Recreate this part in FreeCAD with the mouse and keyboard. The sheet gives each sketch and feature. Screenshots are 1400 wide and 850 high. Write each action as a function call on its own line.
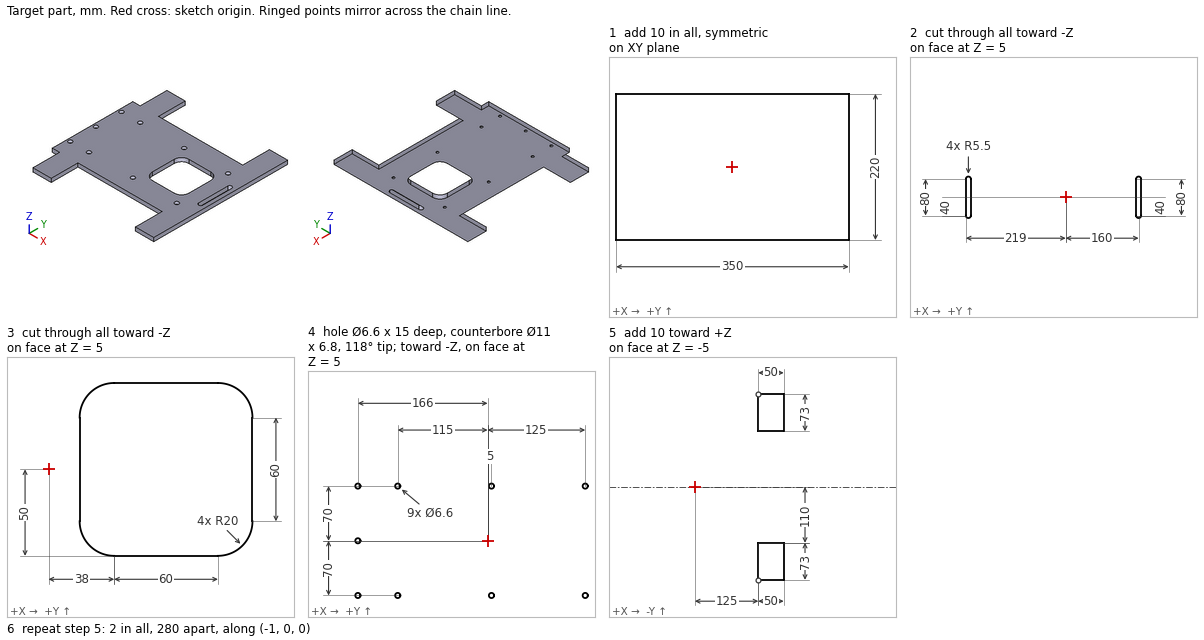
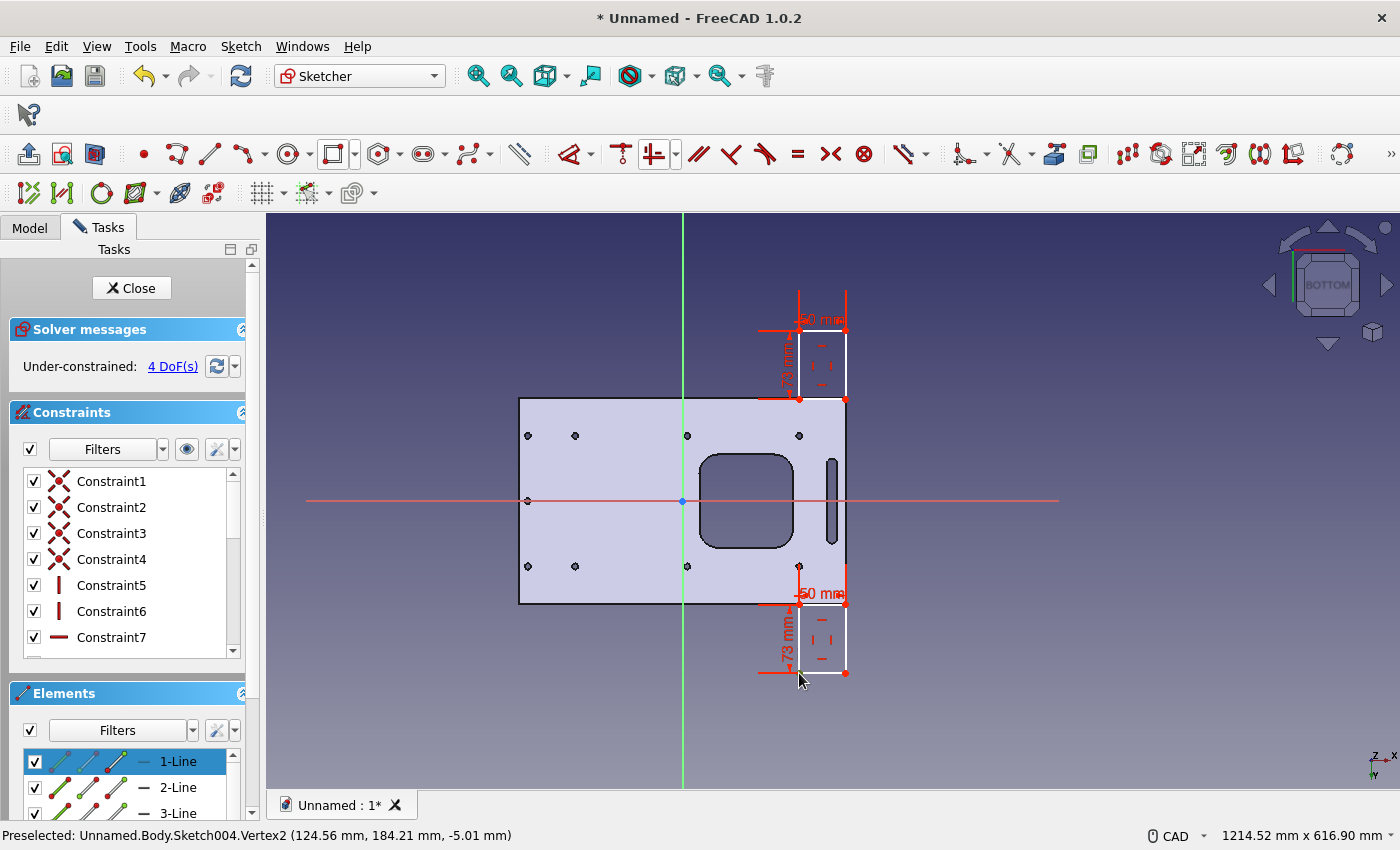
click(799, 331)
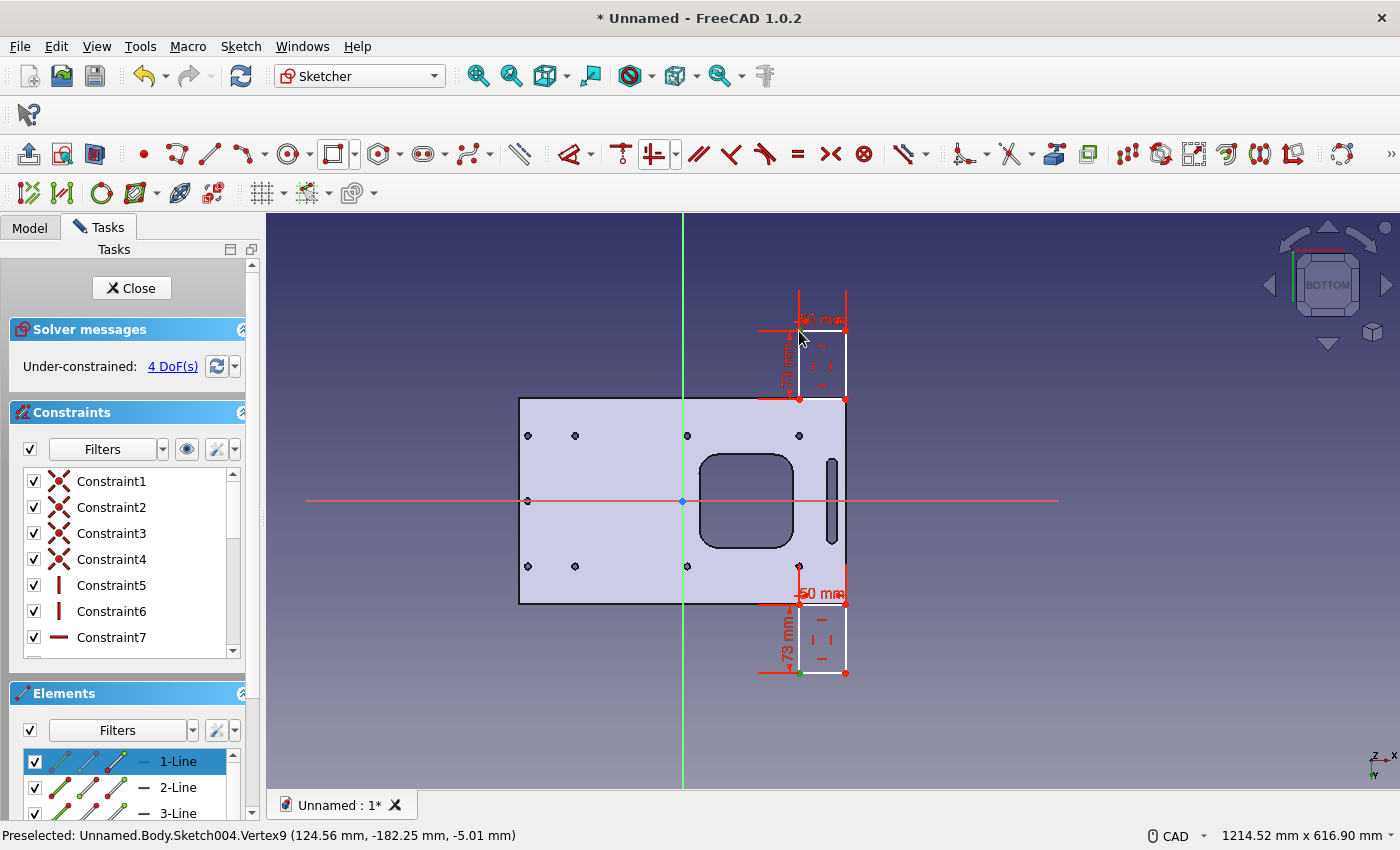
click(361, 501)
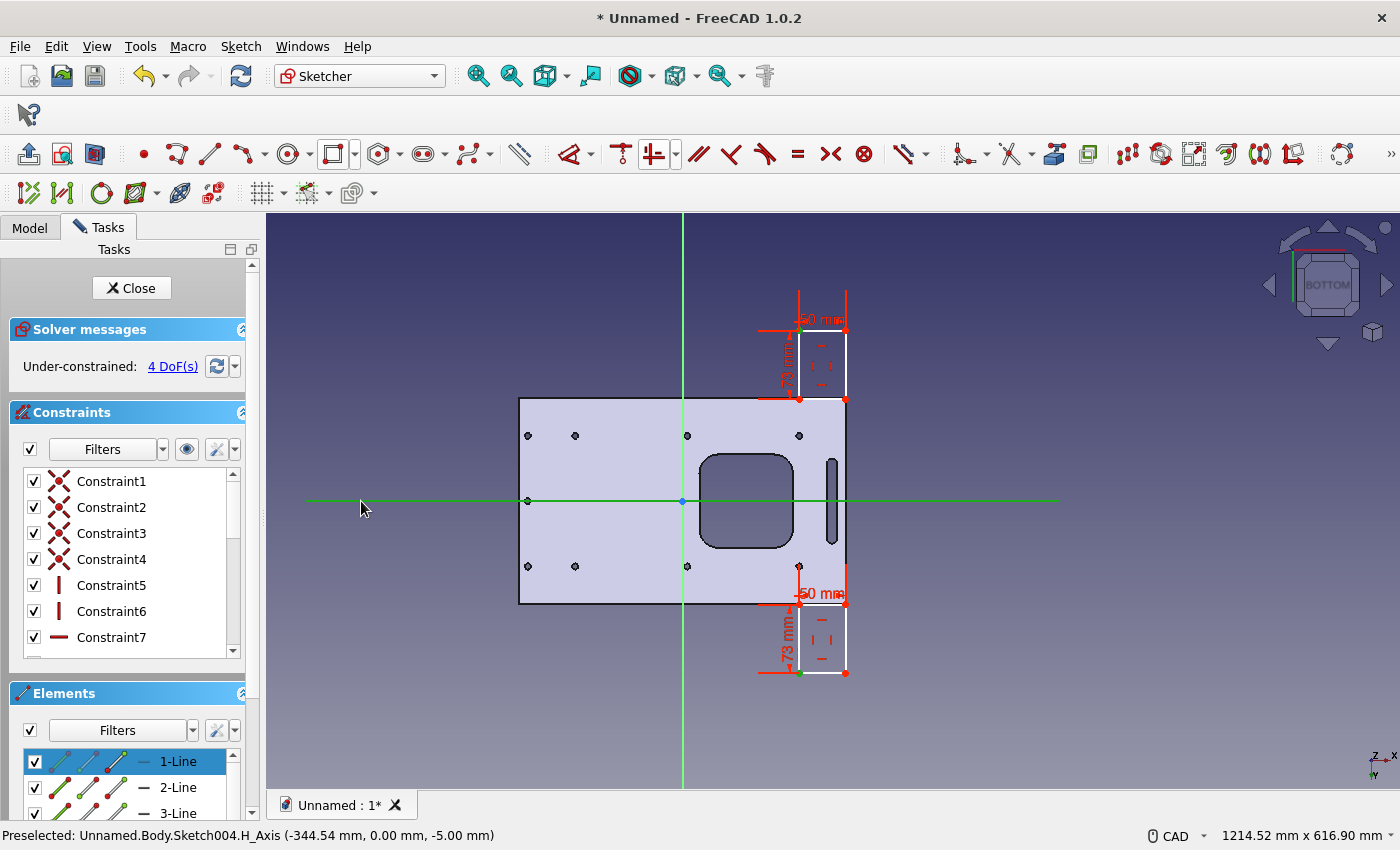
key(s)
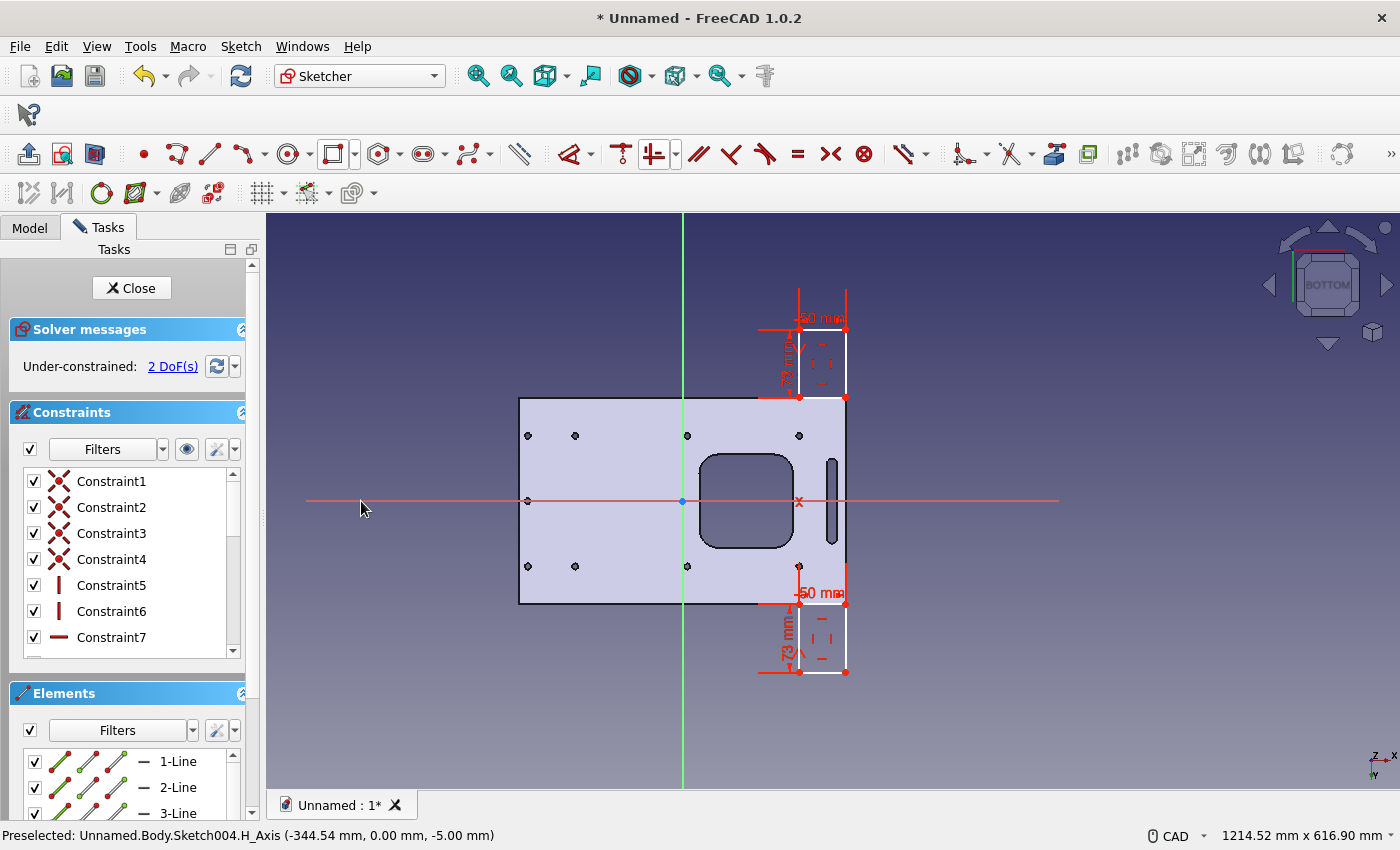
click(568, 154)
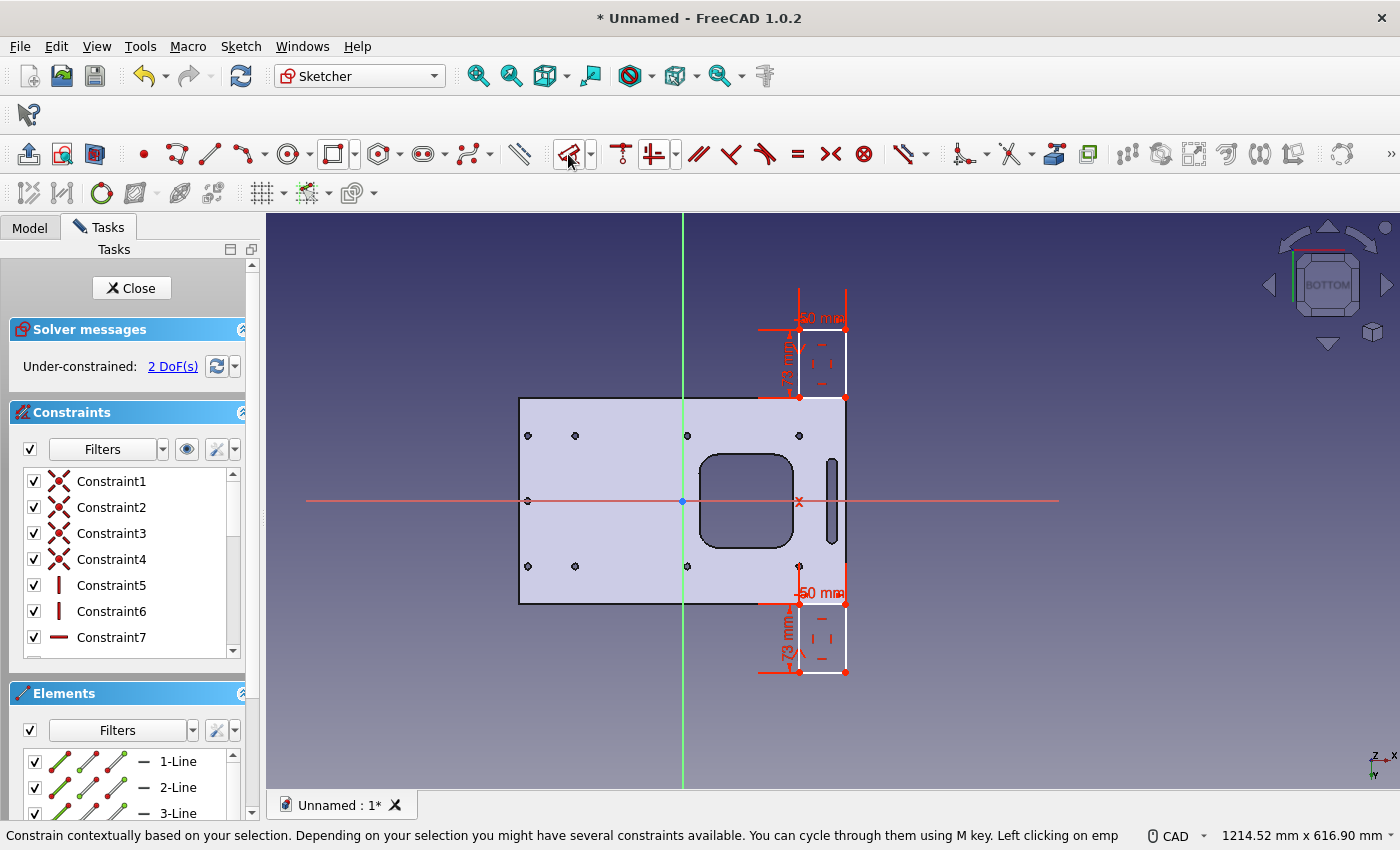
click(799, 604)
click(741, 638)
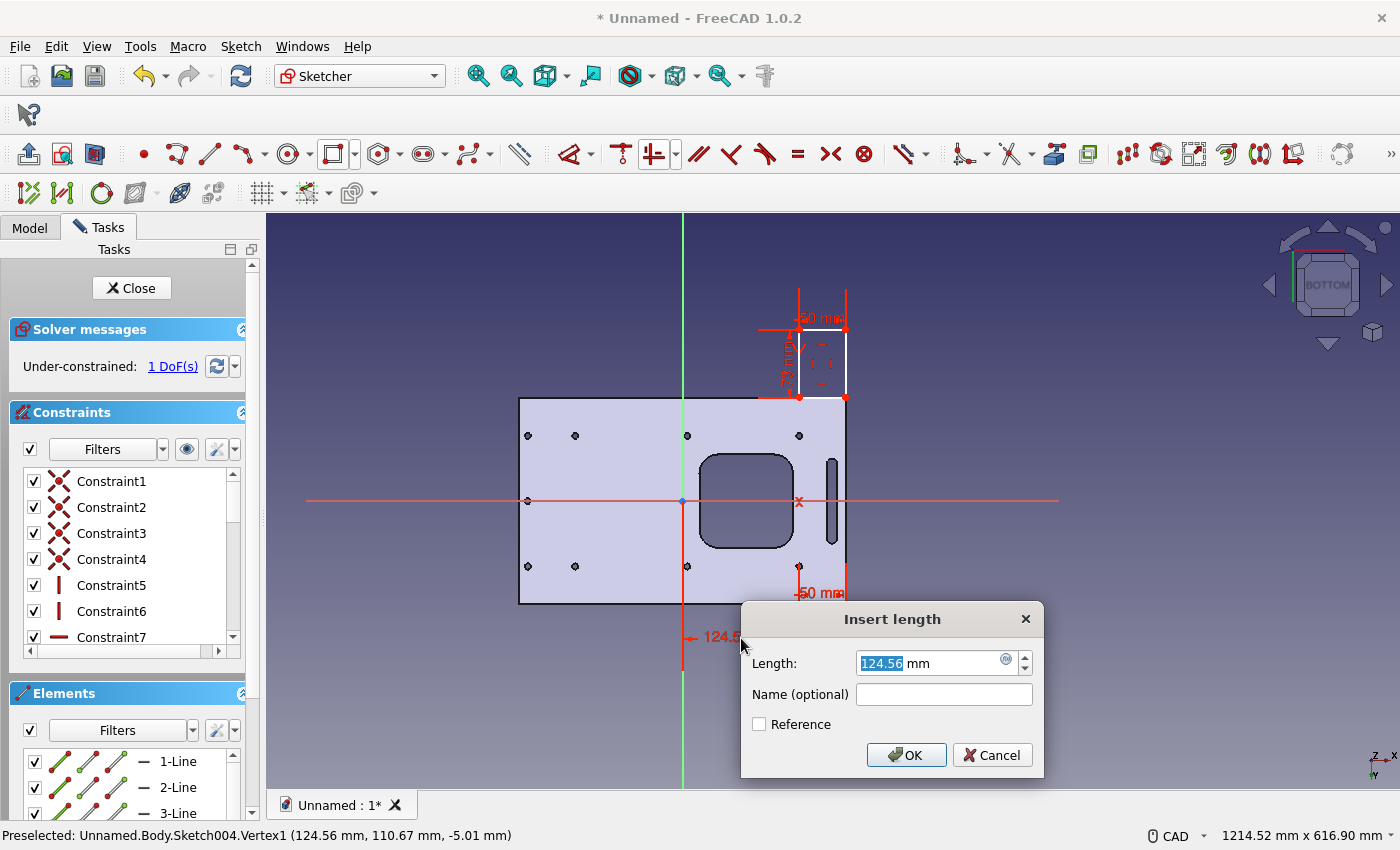
text(125)
key(Return)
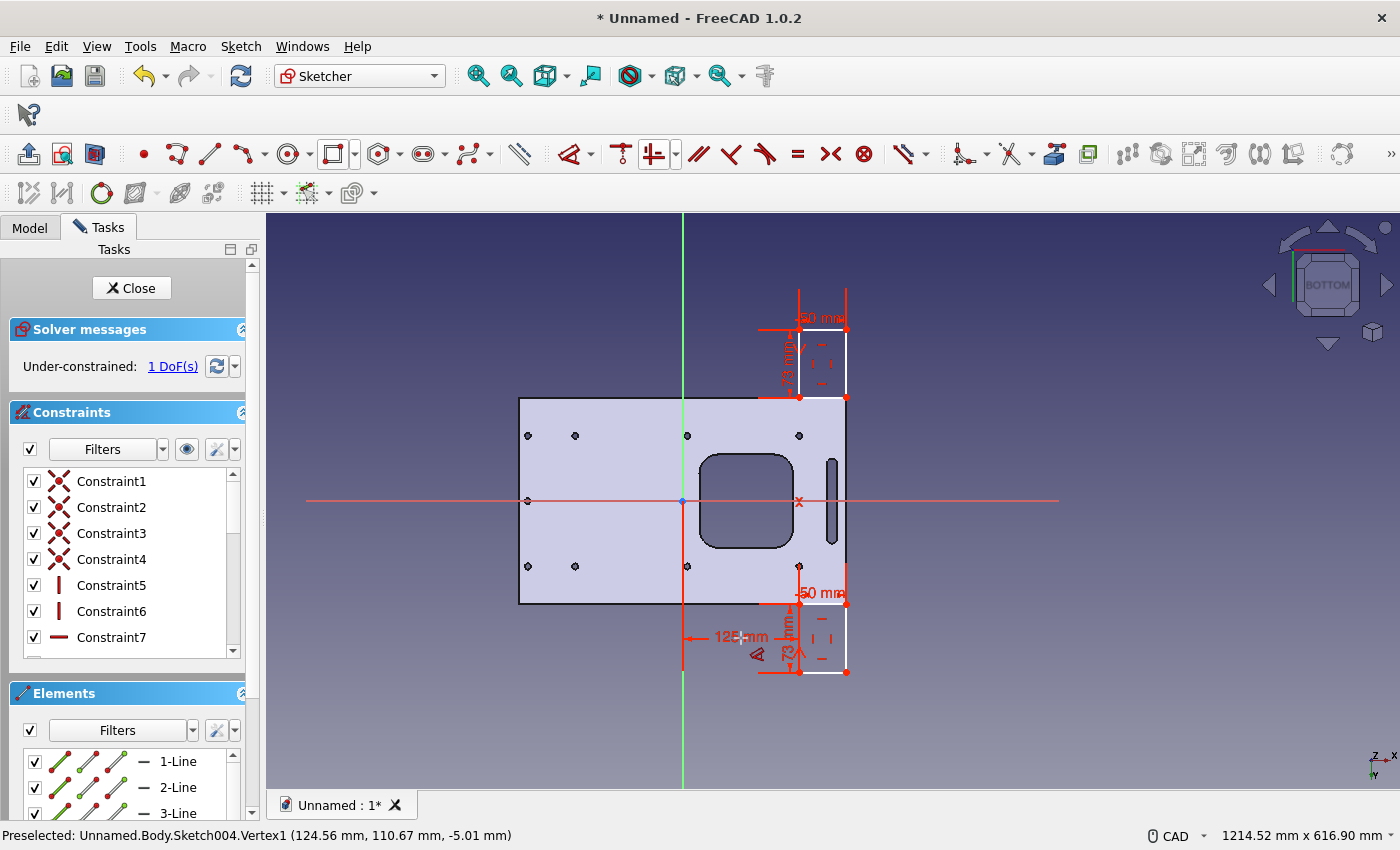
click(799, 604)
click(649, 553)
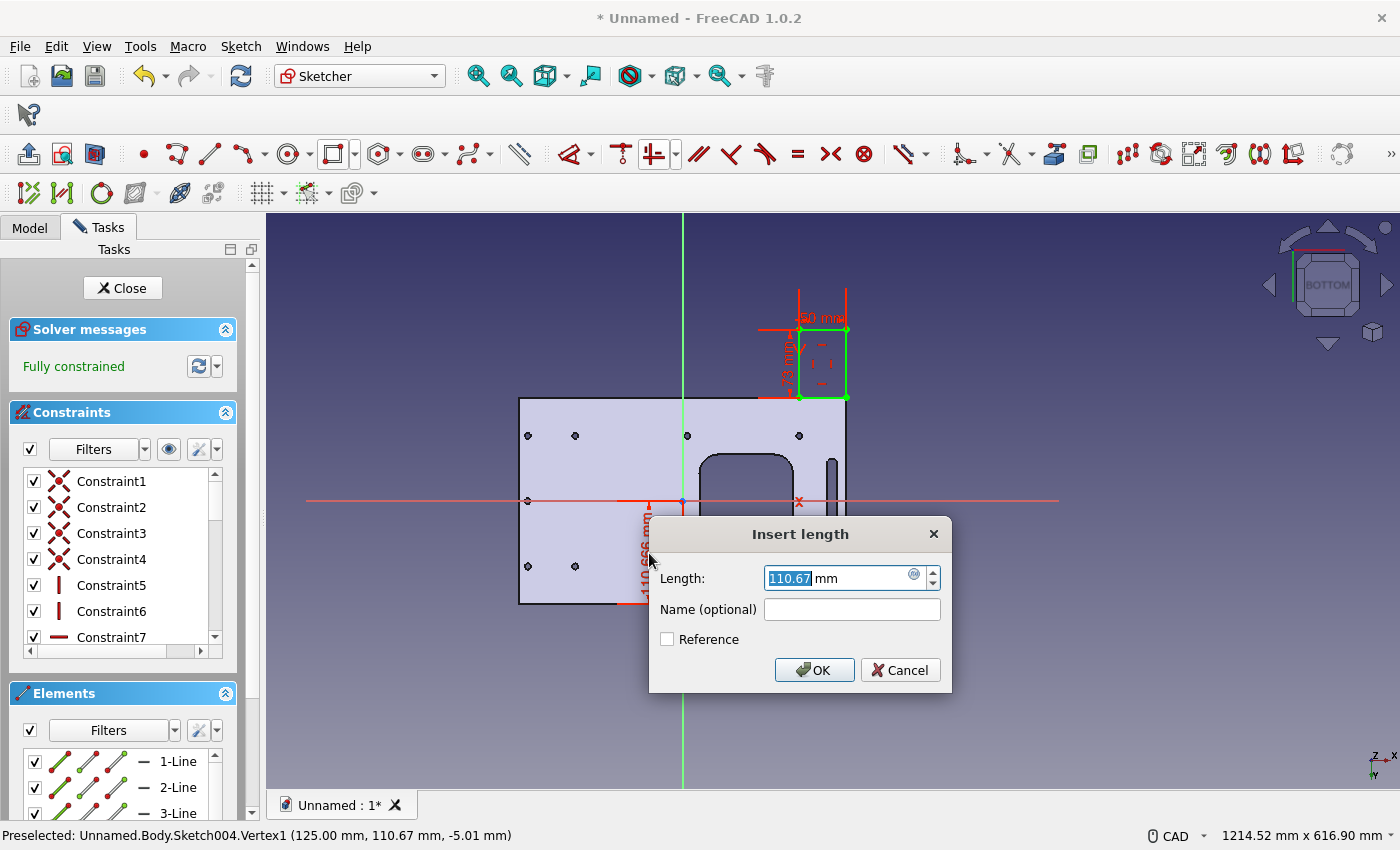
text(110)
key(Return)
key(Escape)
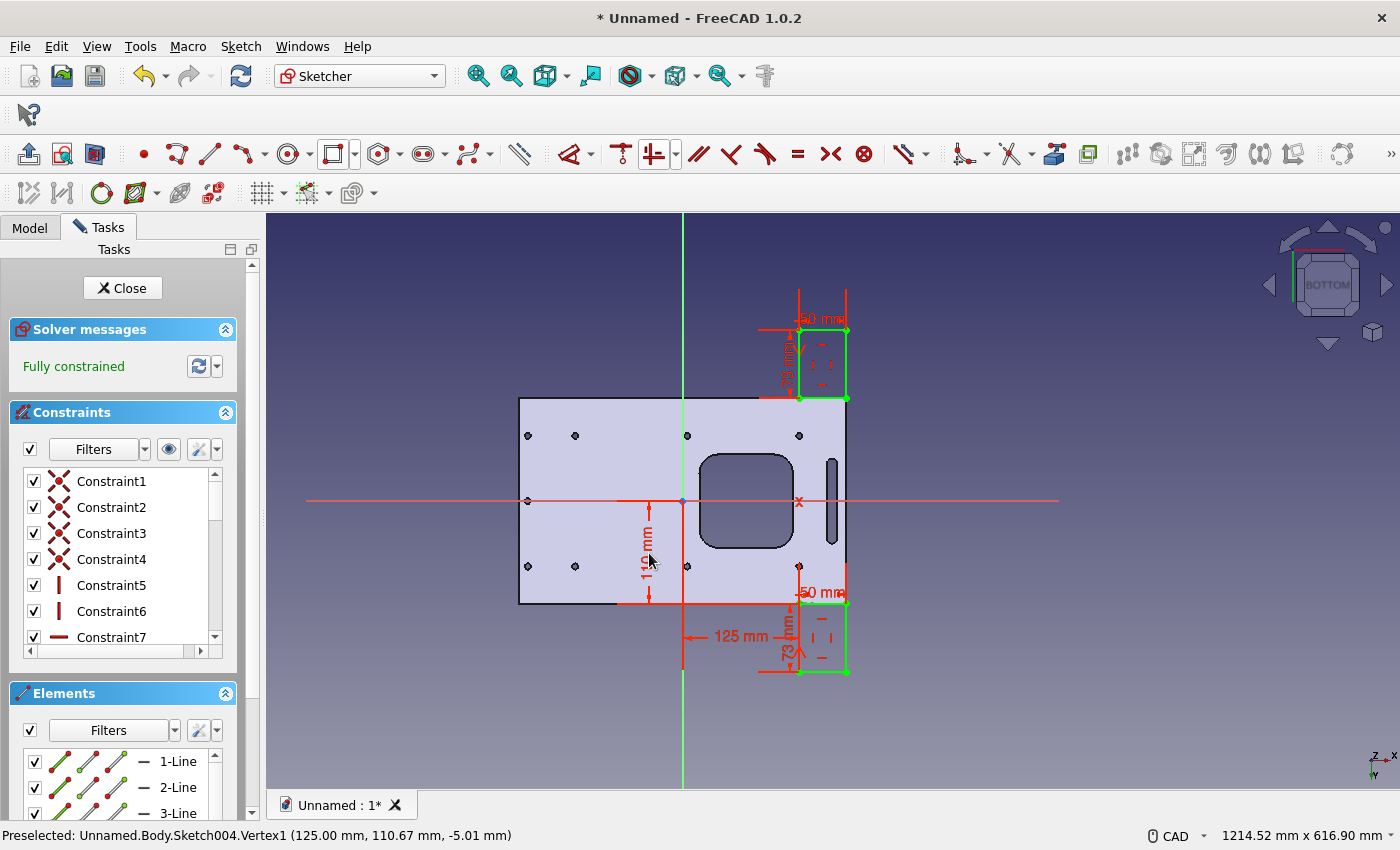
click(123, 288)